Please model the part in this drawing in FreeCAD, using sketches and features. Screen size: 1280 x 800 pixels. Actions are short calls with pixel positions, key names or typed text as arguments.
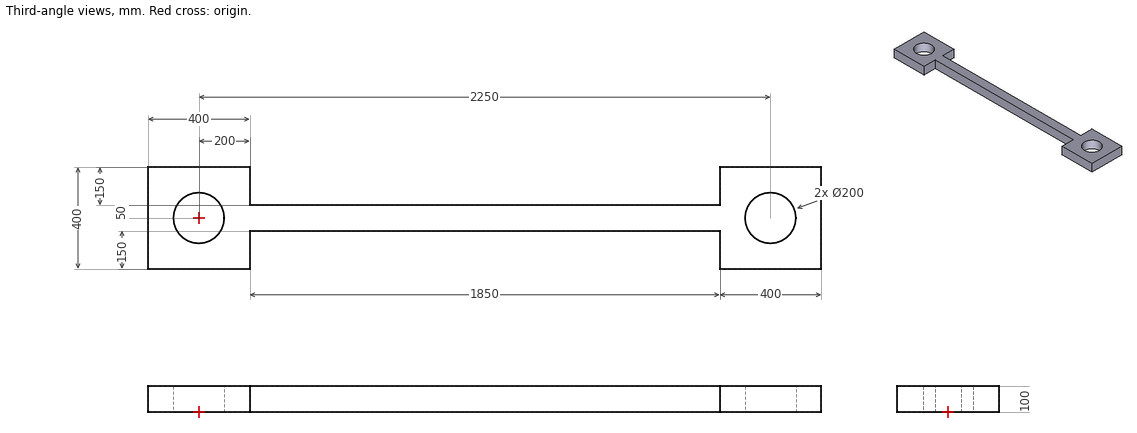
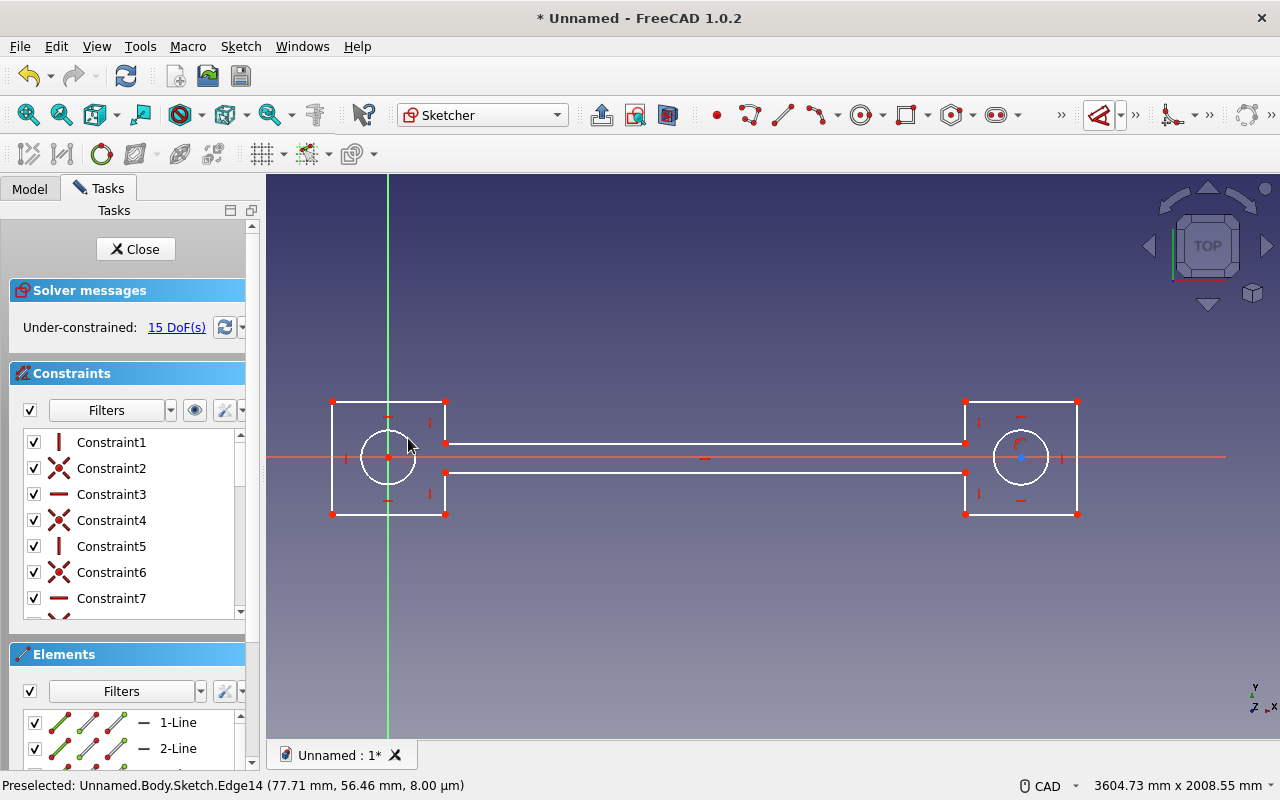
click(1040, 438)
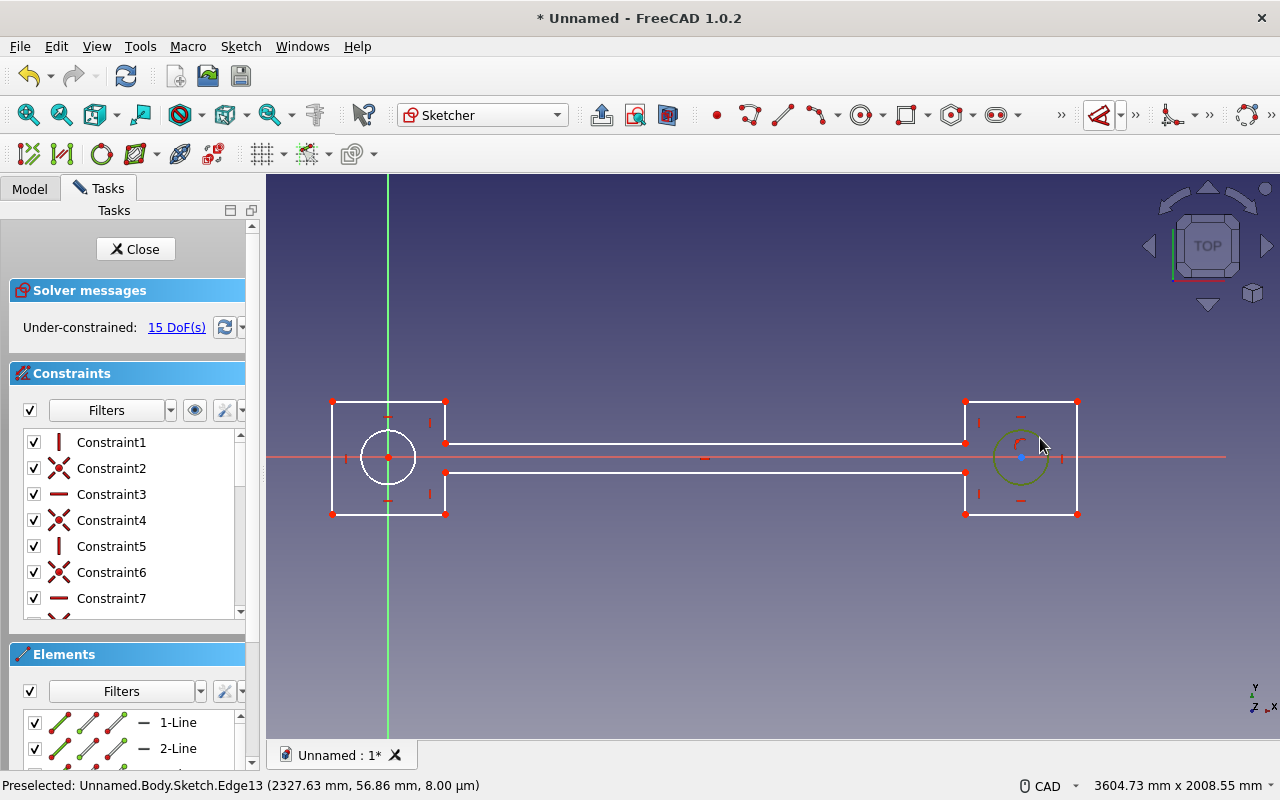
click(407, 438)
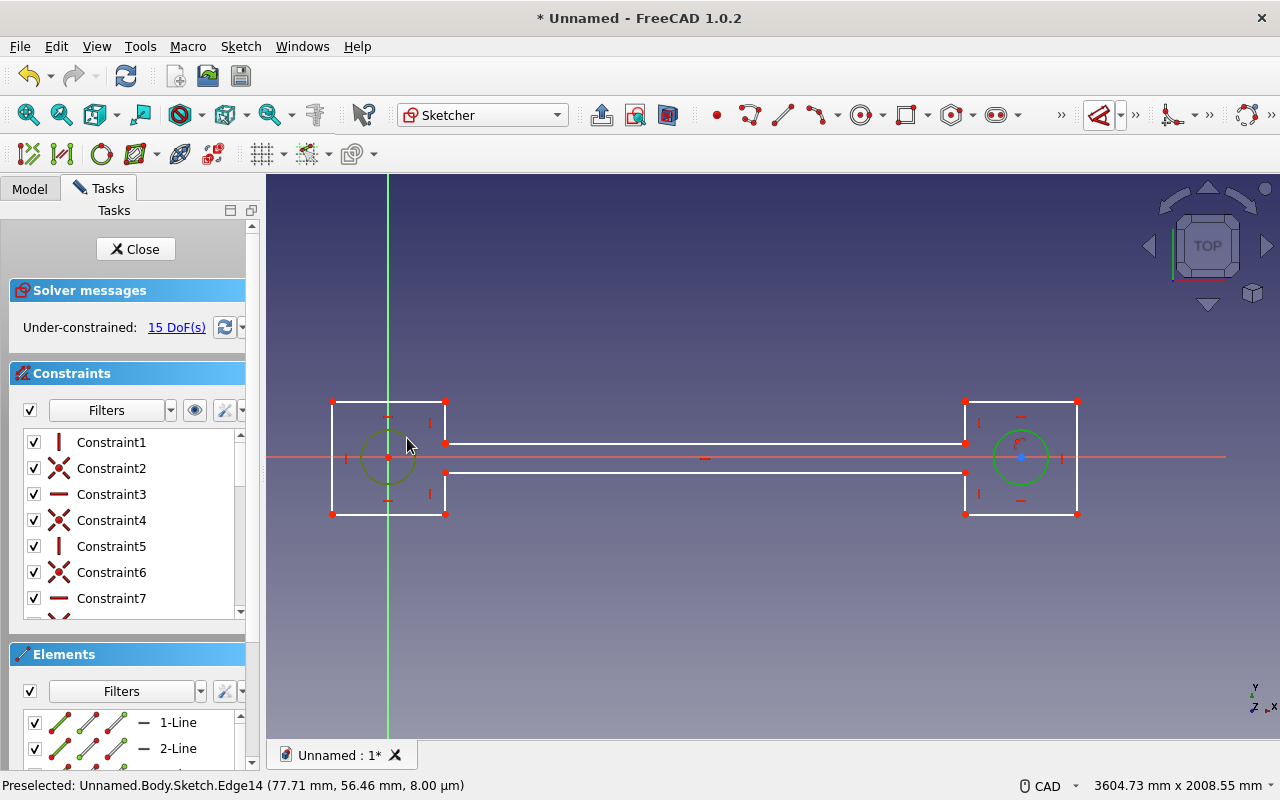
key(e)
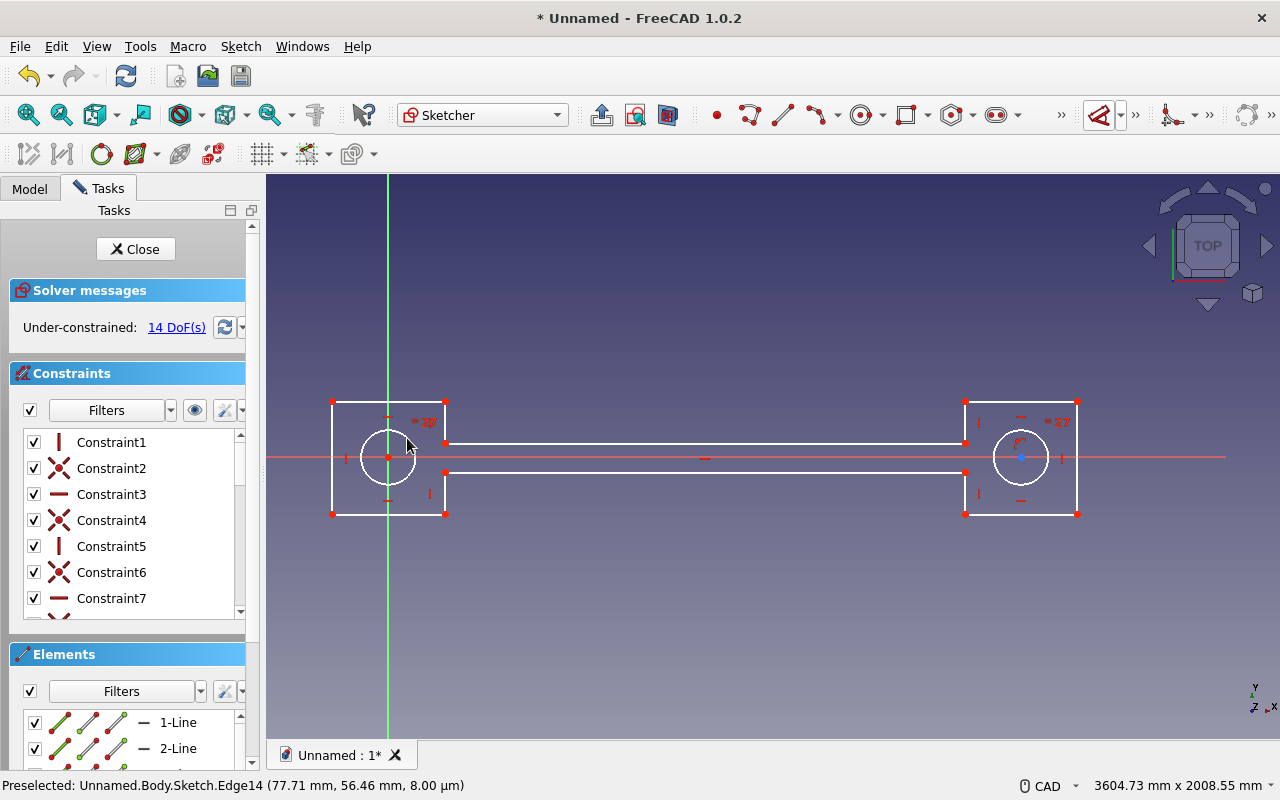
click(1098, 116)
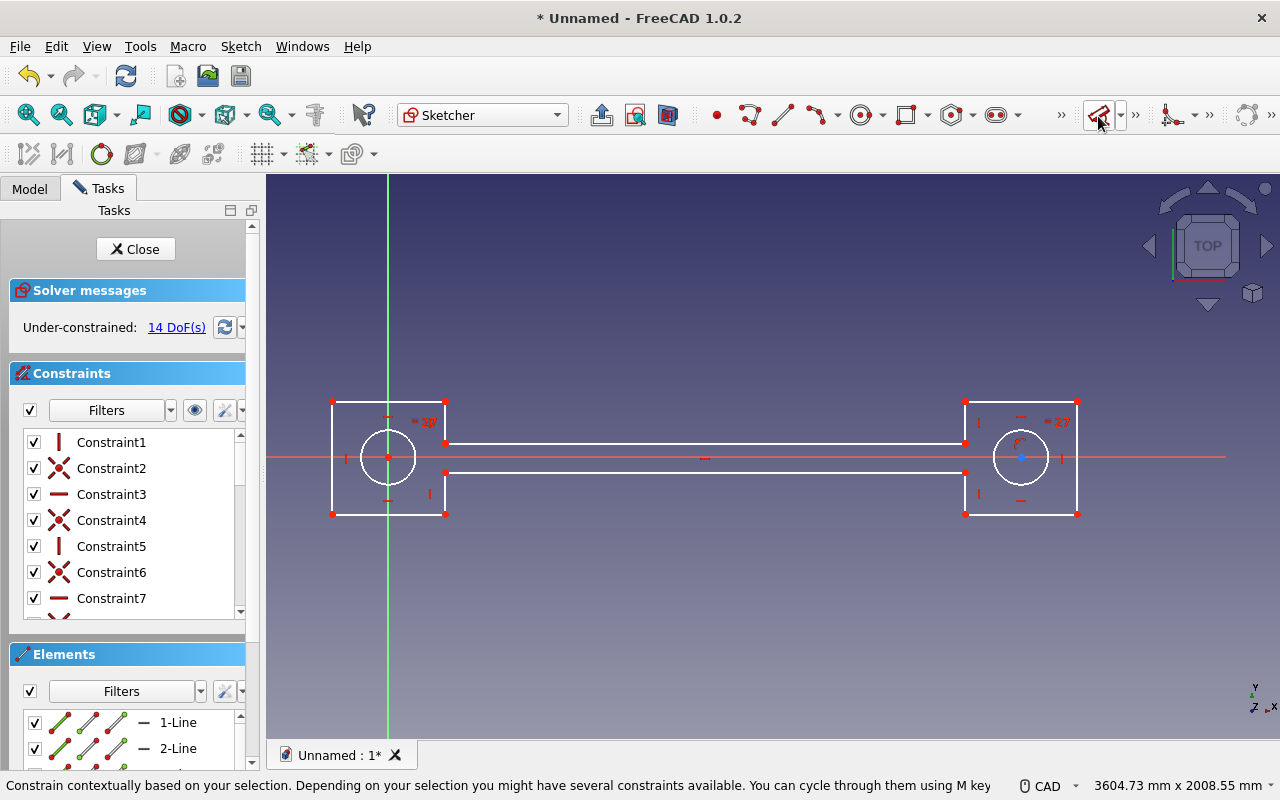
click(1040, 438)
click(1062, 415)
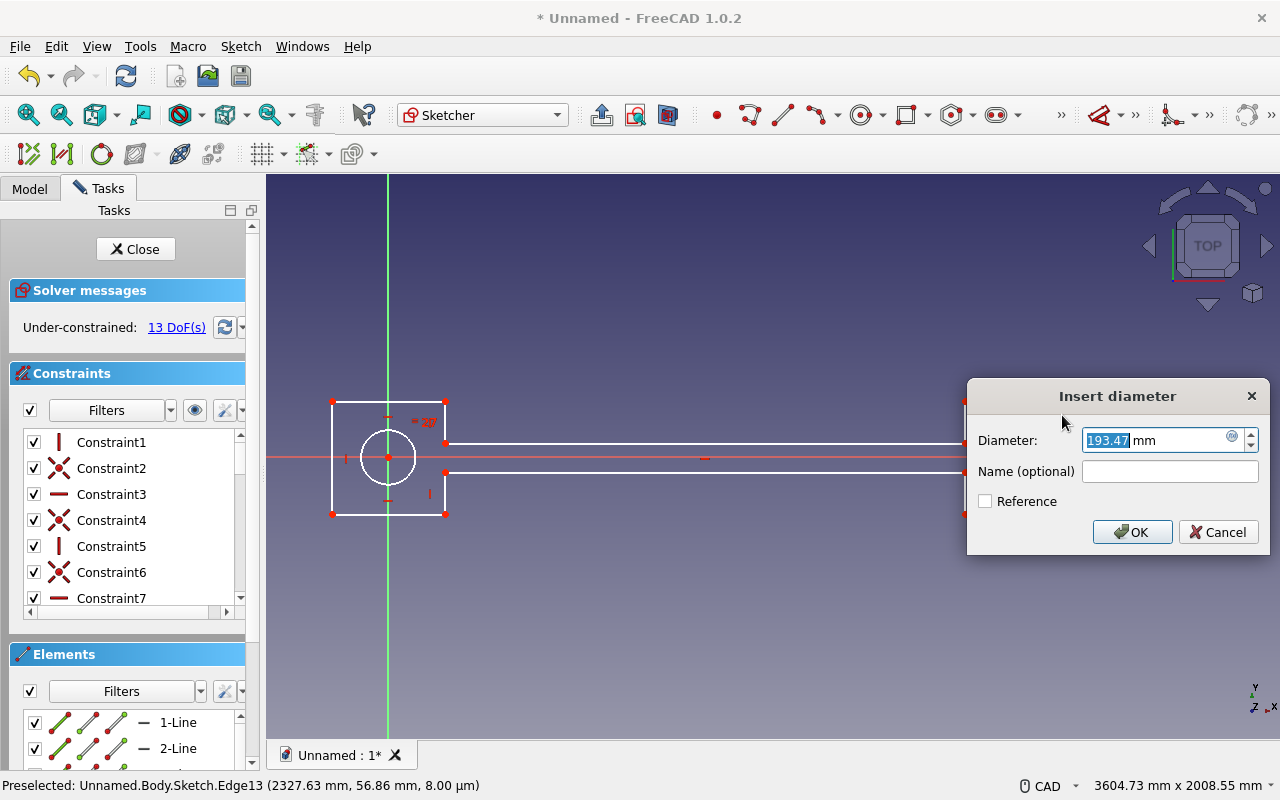
text(200)
key(Return)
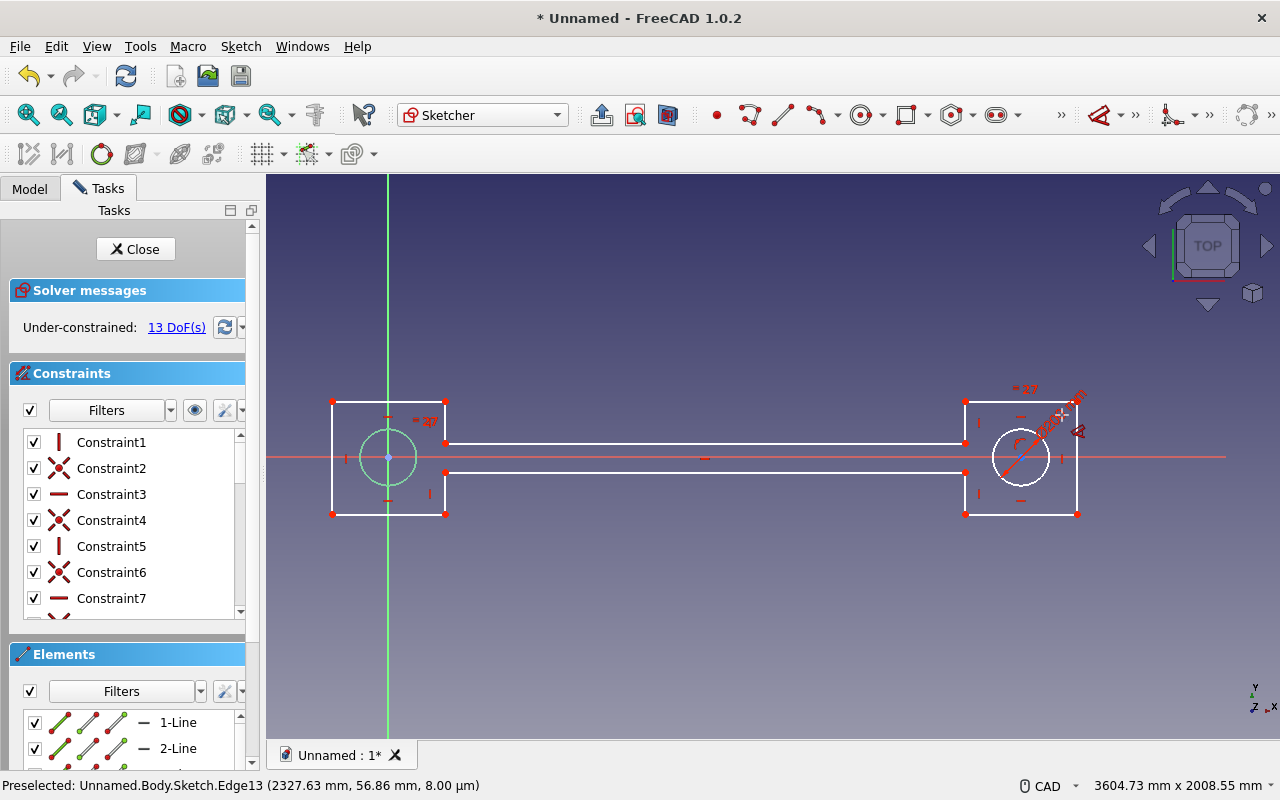
click(445, 431)
click(411, 423)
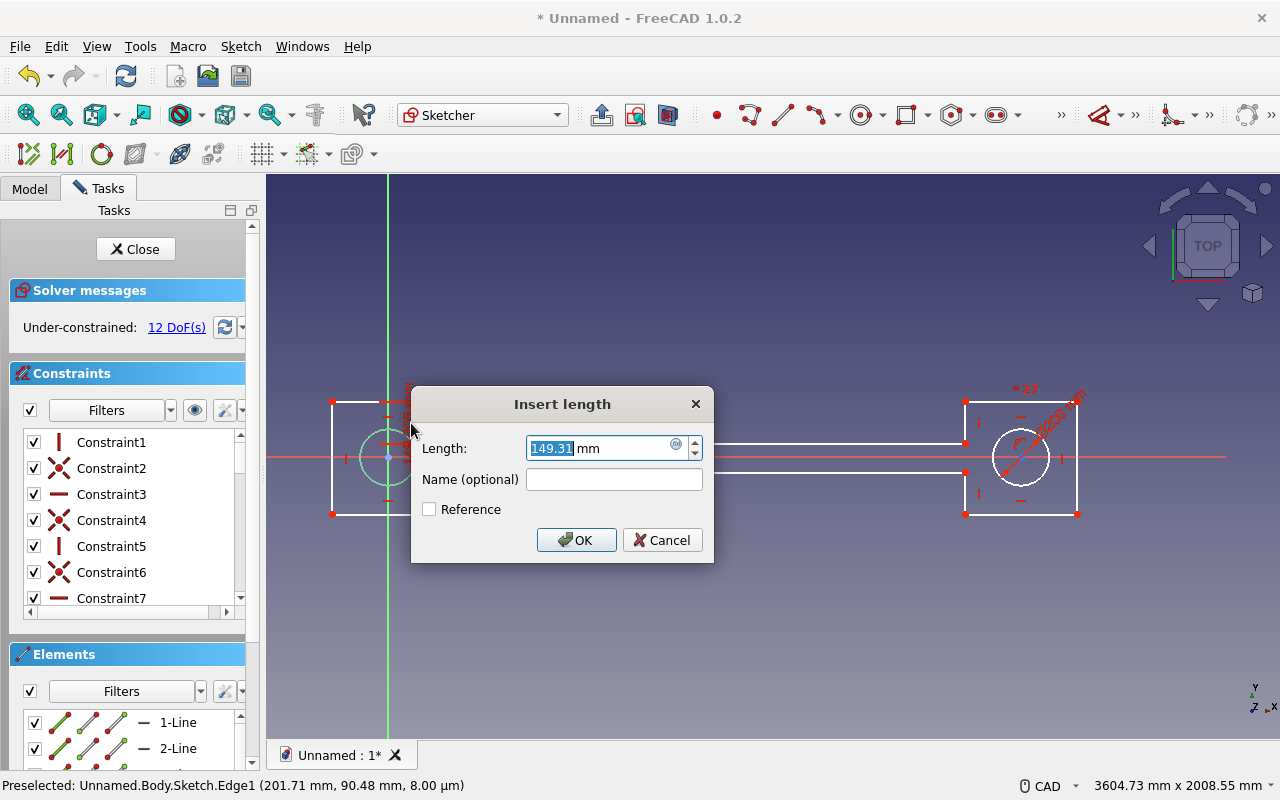
text(150)
key(Return)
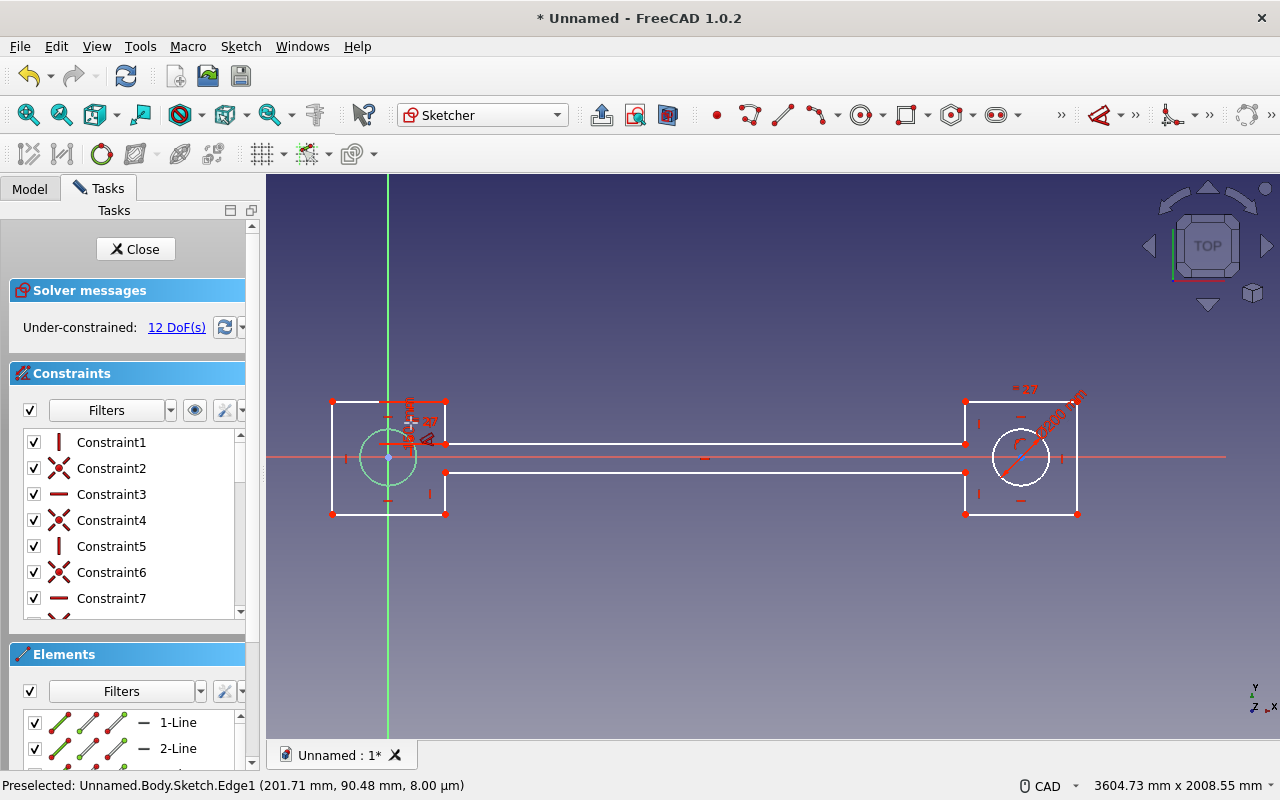
click(411, 402)
click(363, 368)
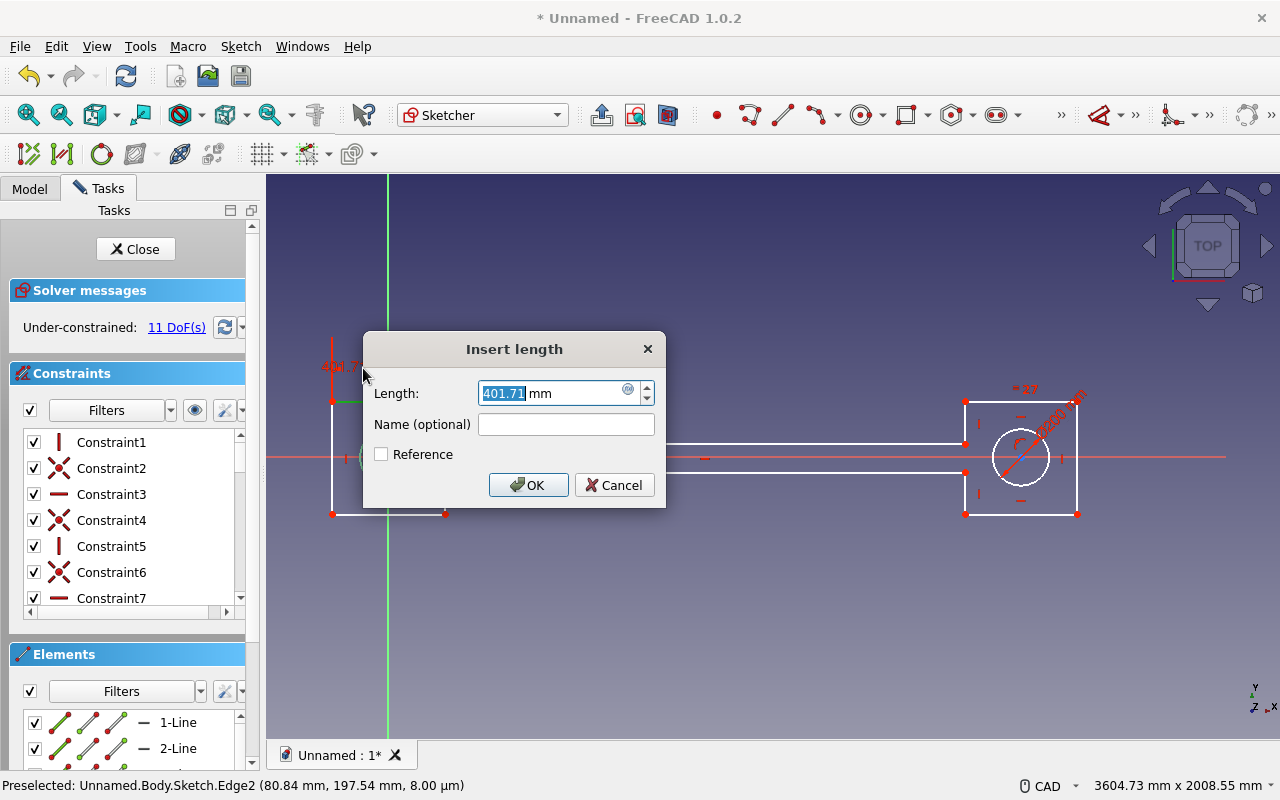
text(400)
key(Return)